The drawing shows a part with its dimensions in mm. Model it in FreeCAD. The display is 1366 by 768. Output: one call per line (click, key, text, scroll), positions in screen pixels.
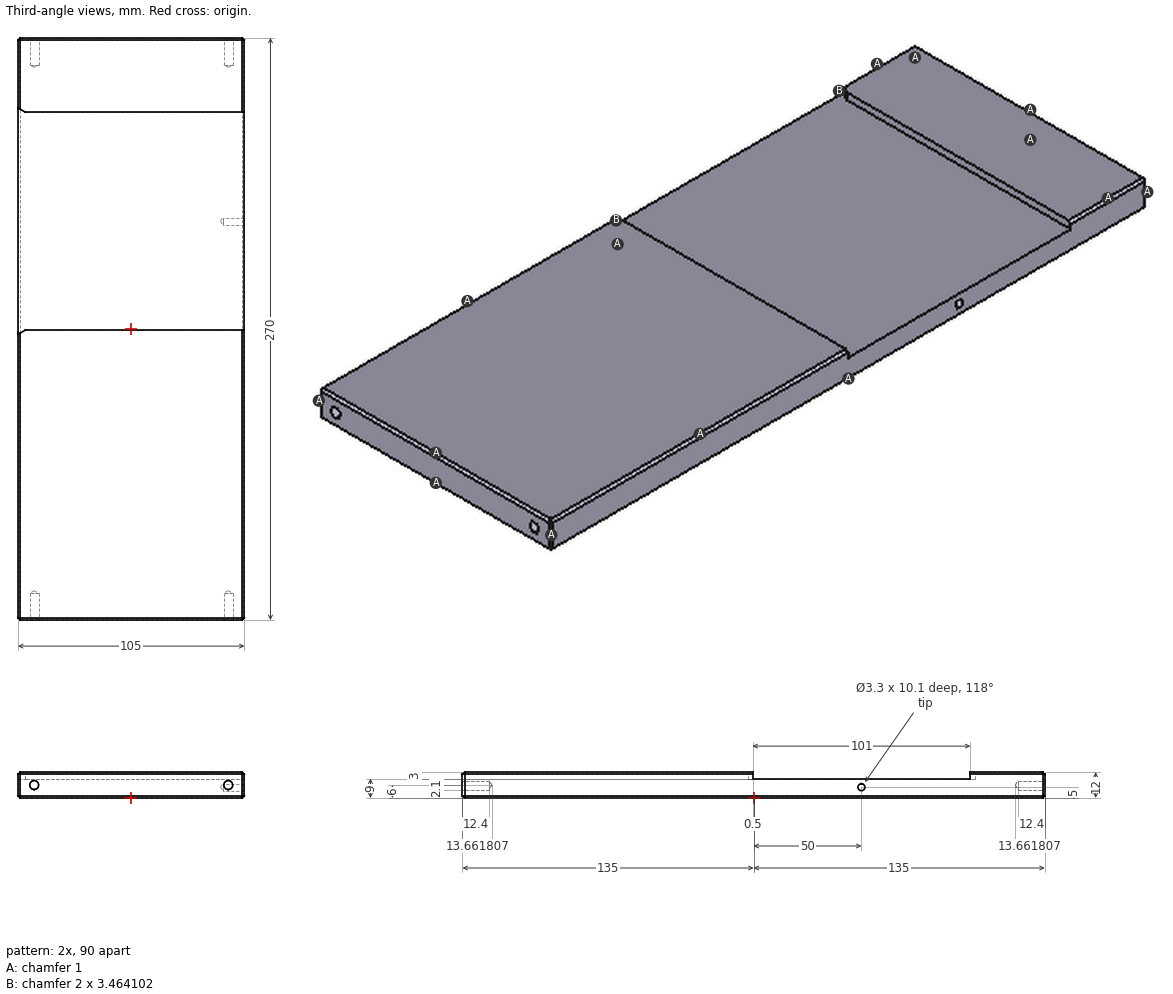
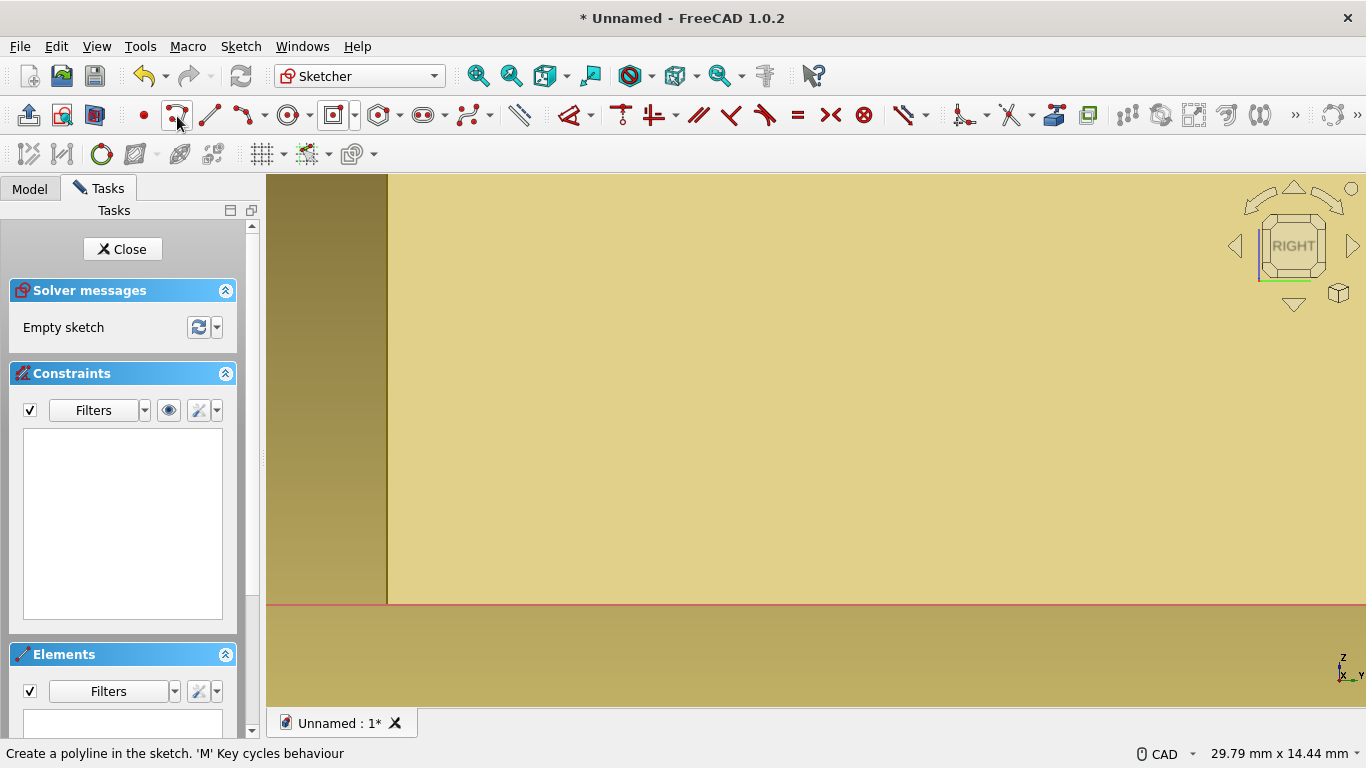
click(892, 383)
click(387, 383)
click(387, 461)
click(845, 461)
click(892, 384)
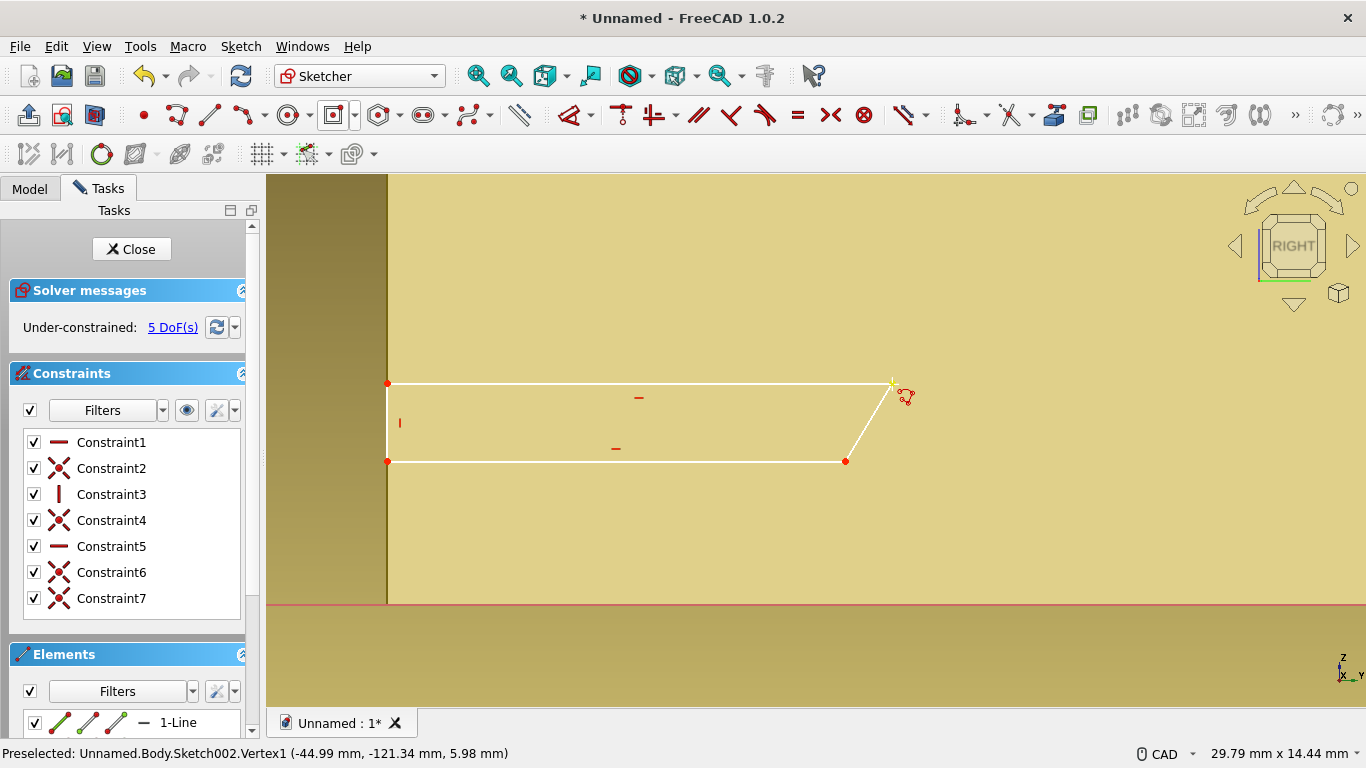
click(210, 116)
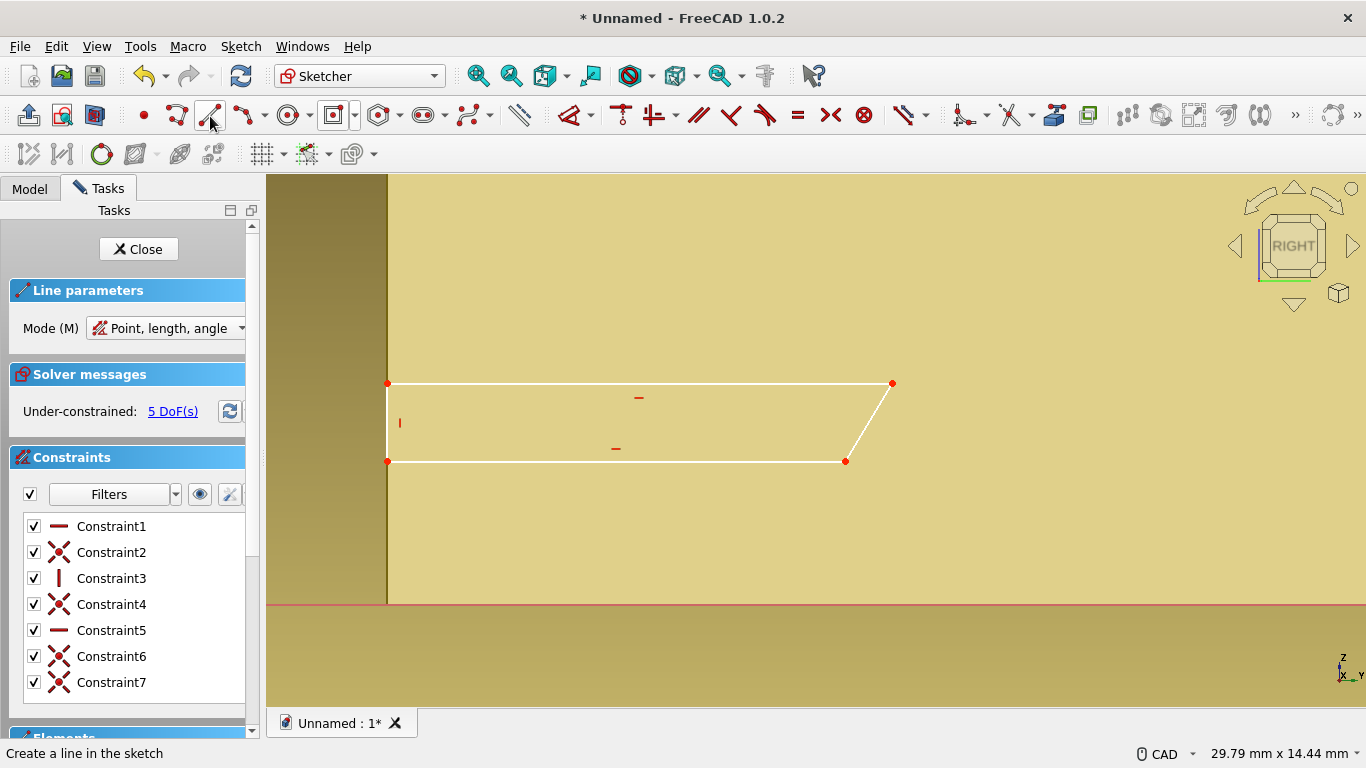
click(942, 383)
click(1094, 383)
key(Escape)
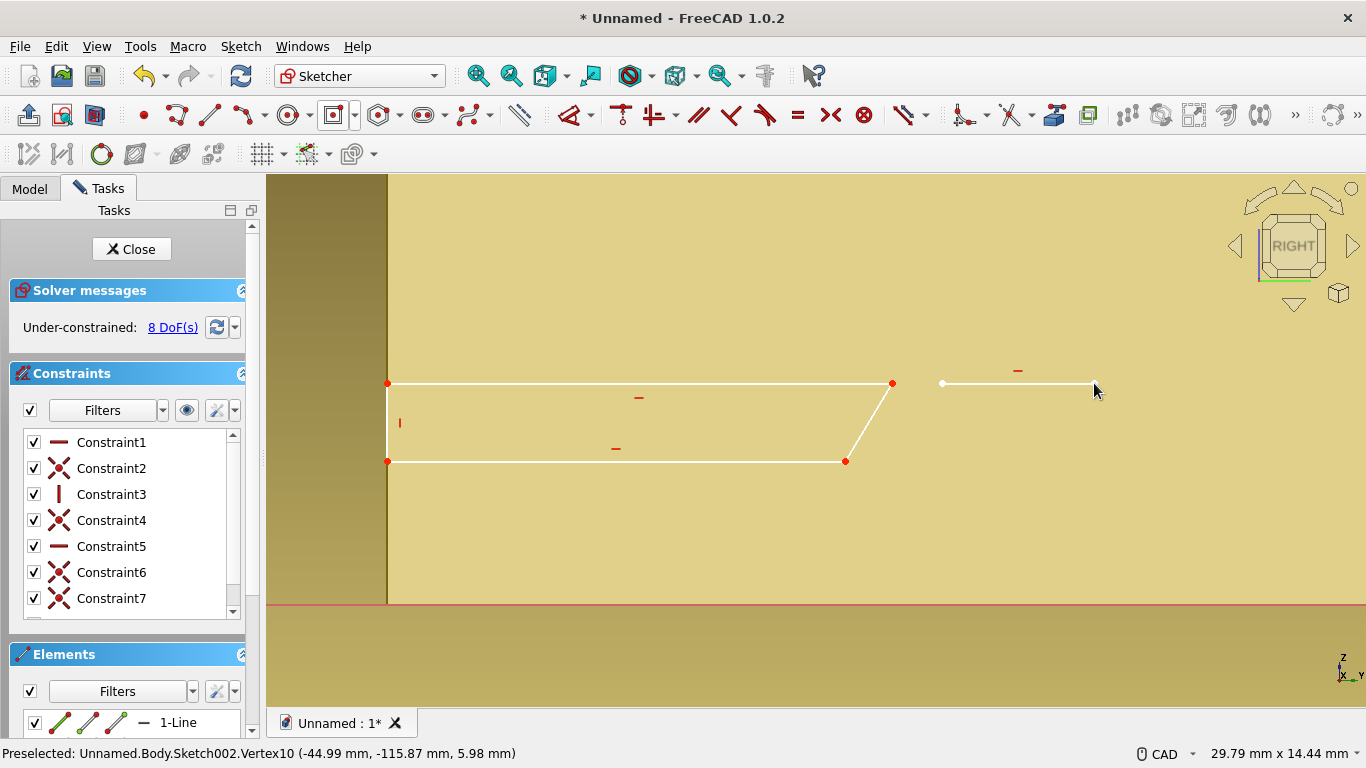
click(988, 384)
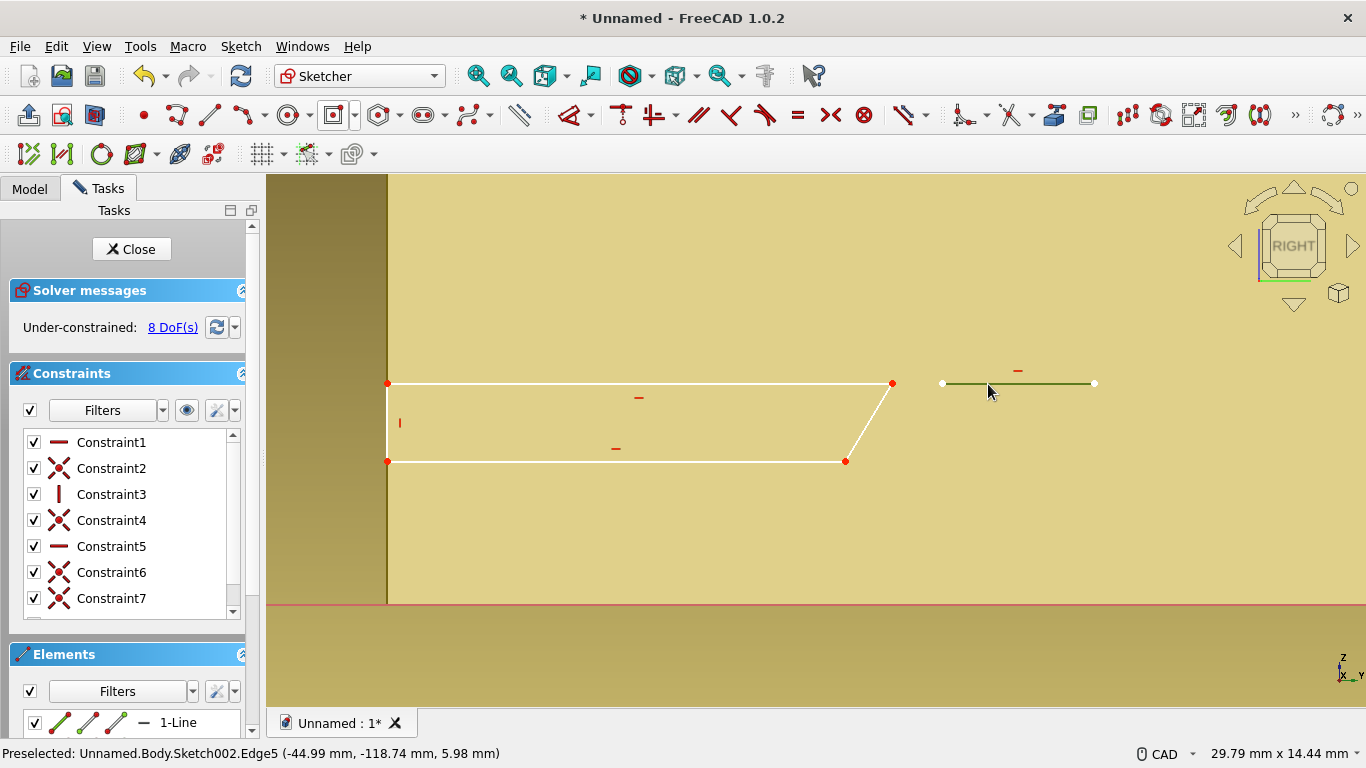
click(520, 116)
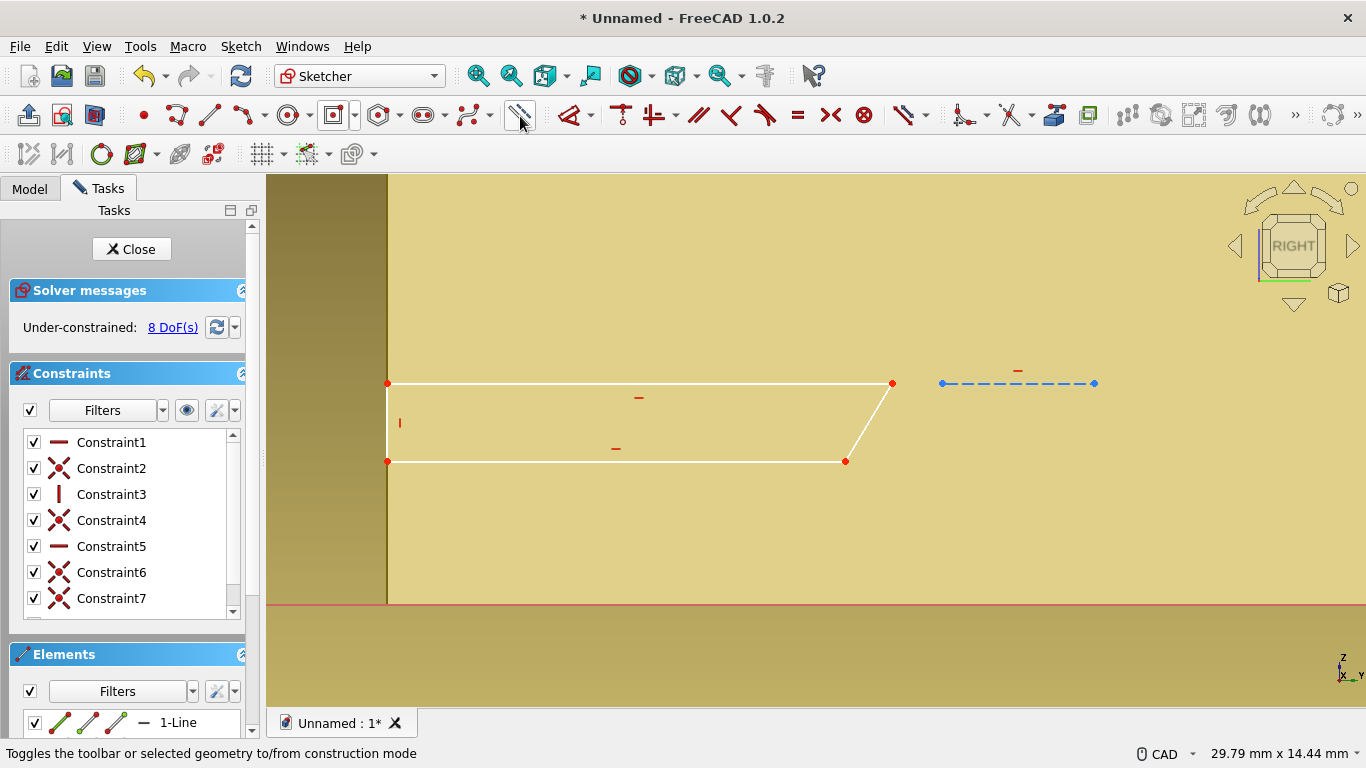
click(568, 116)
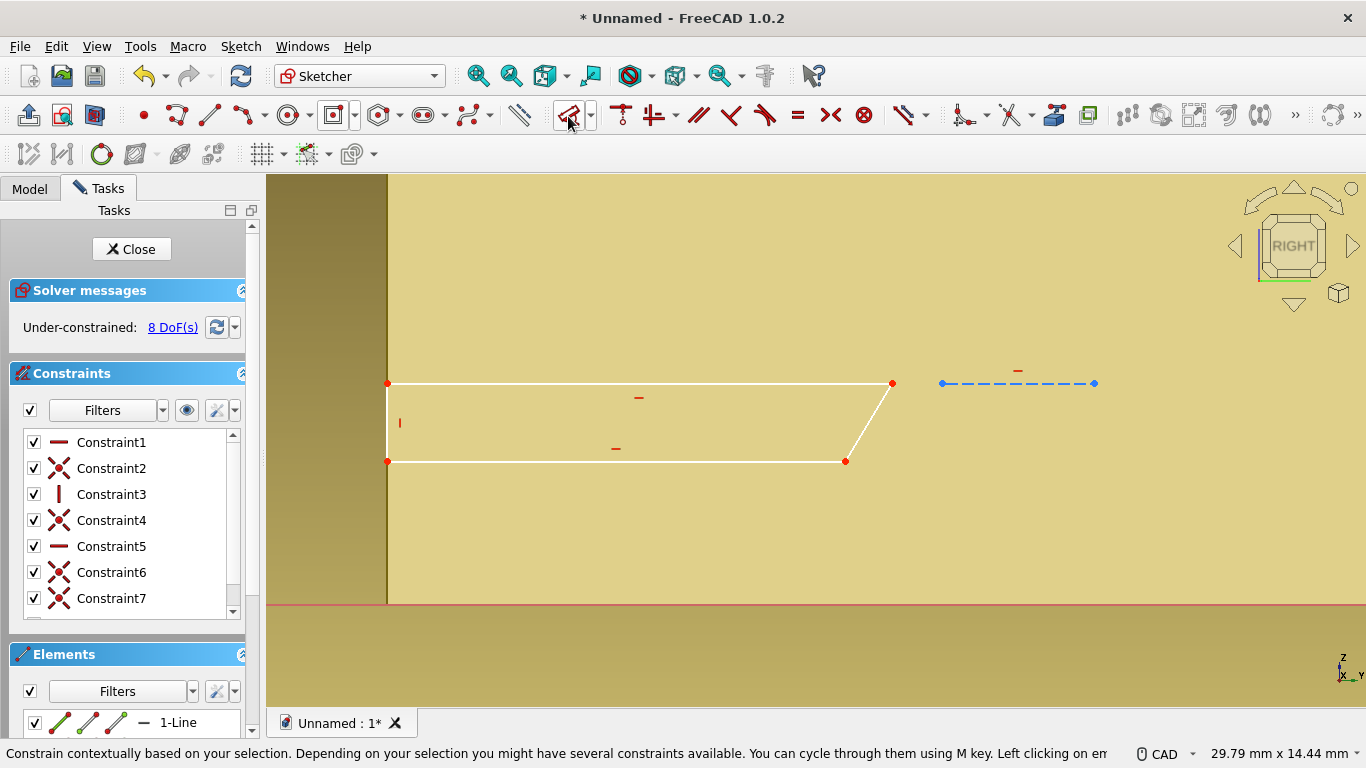
click(892, 384)
click(858, 494)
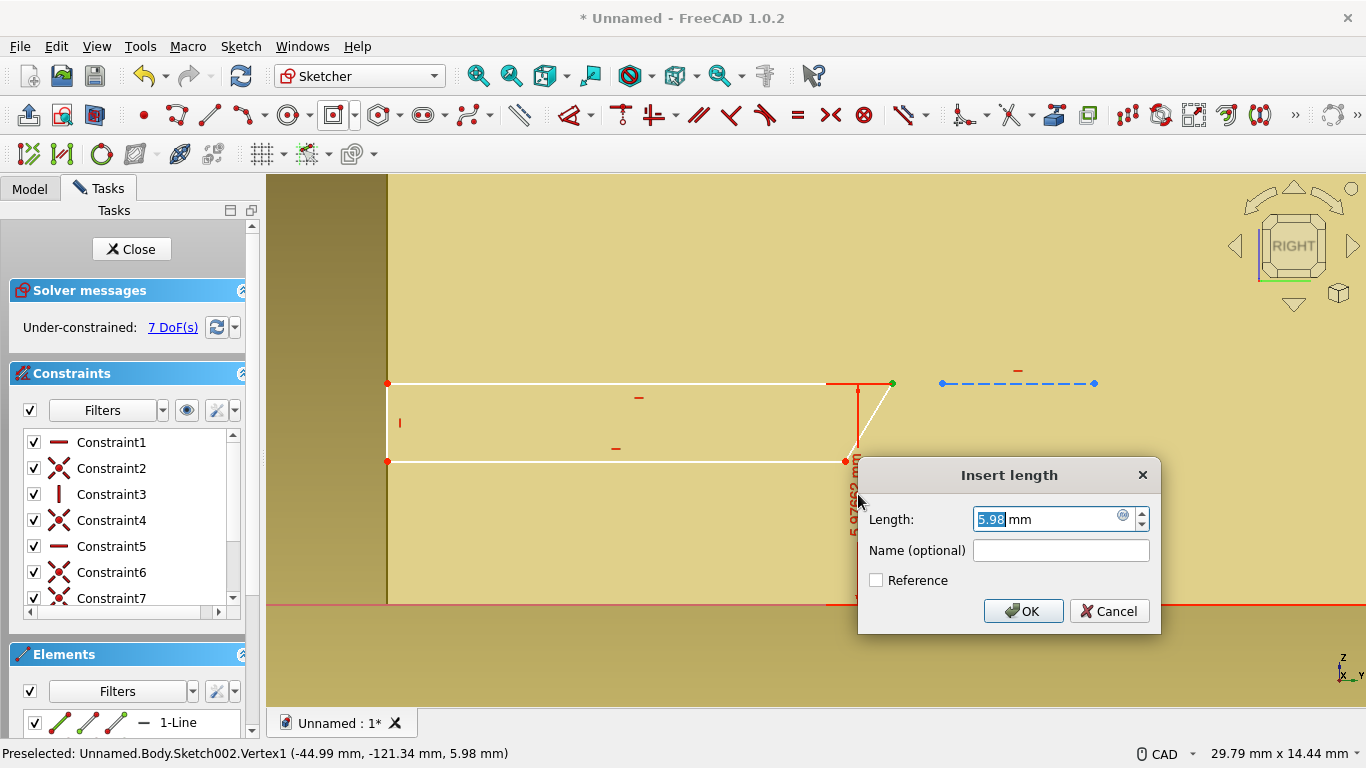
text(6)
key(Return)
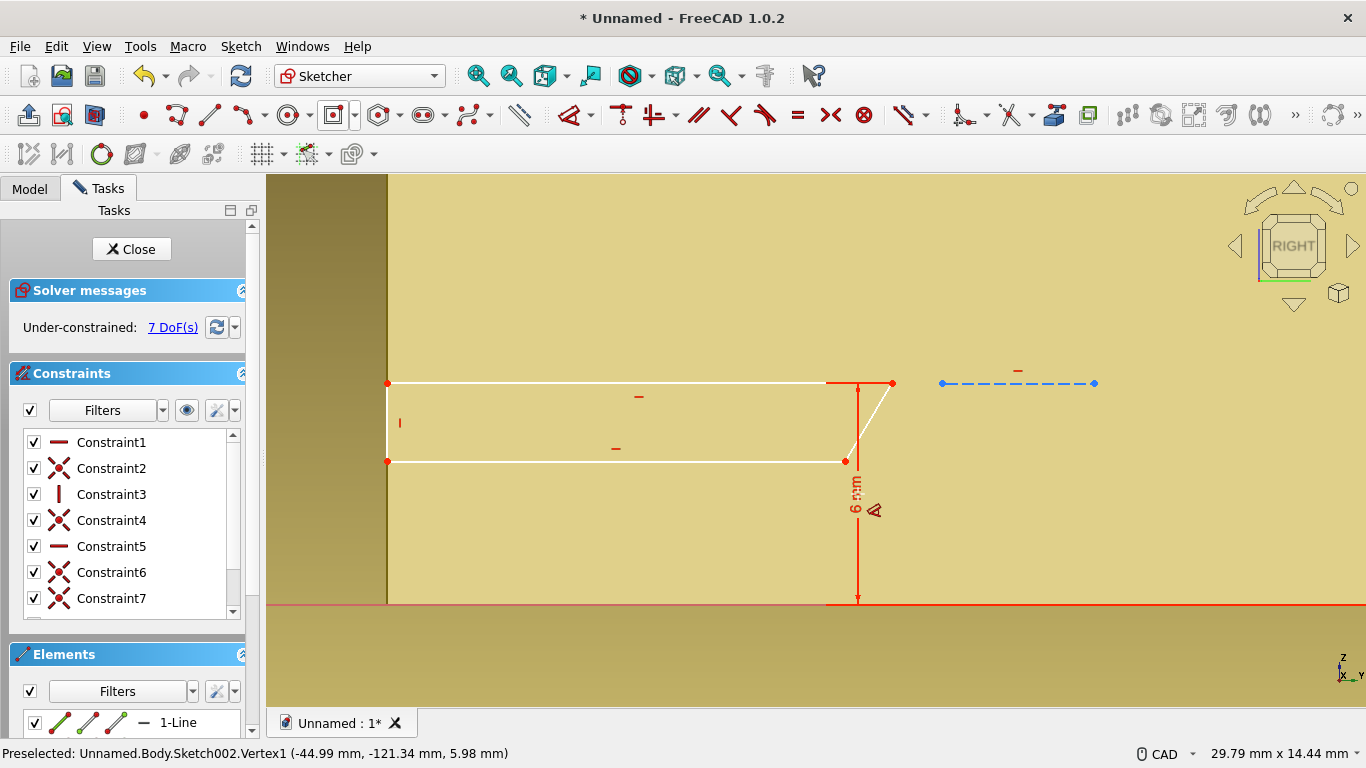
click(942, 384)
click(908, 444)